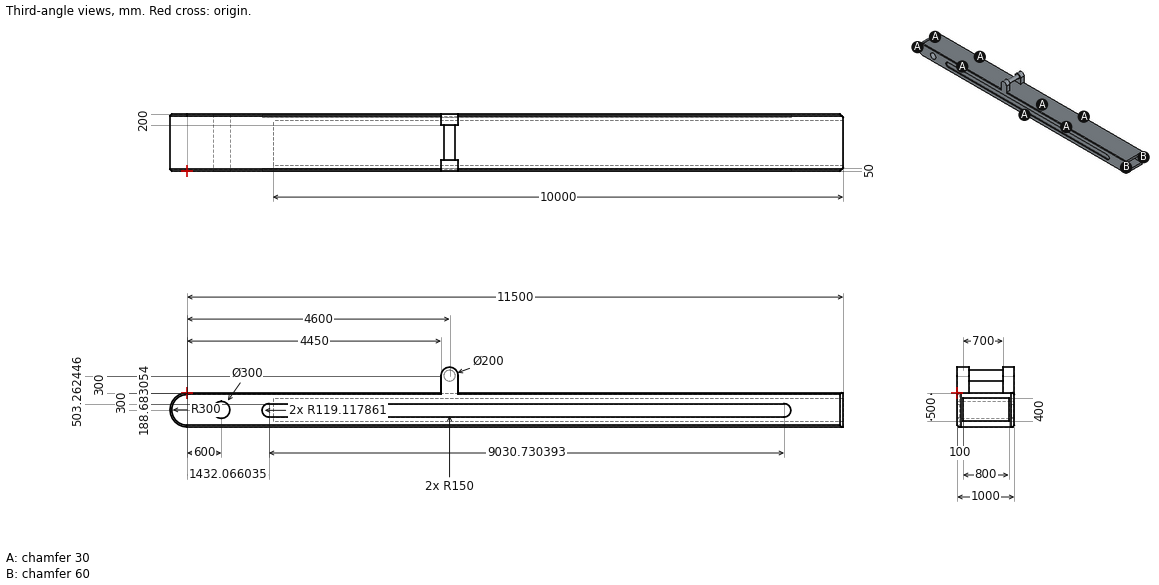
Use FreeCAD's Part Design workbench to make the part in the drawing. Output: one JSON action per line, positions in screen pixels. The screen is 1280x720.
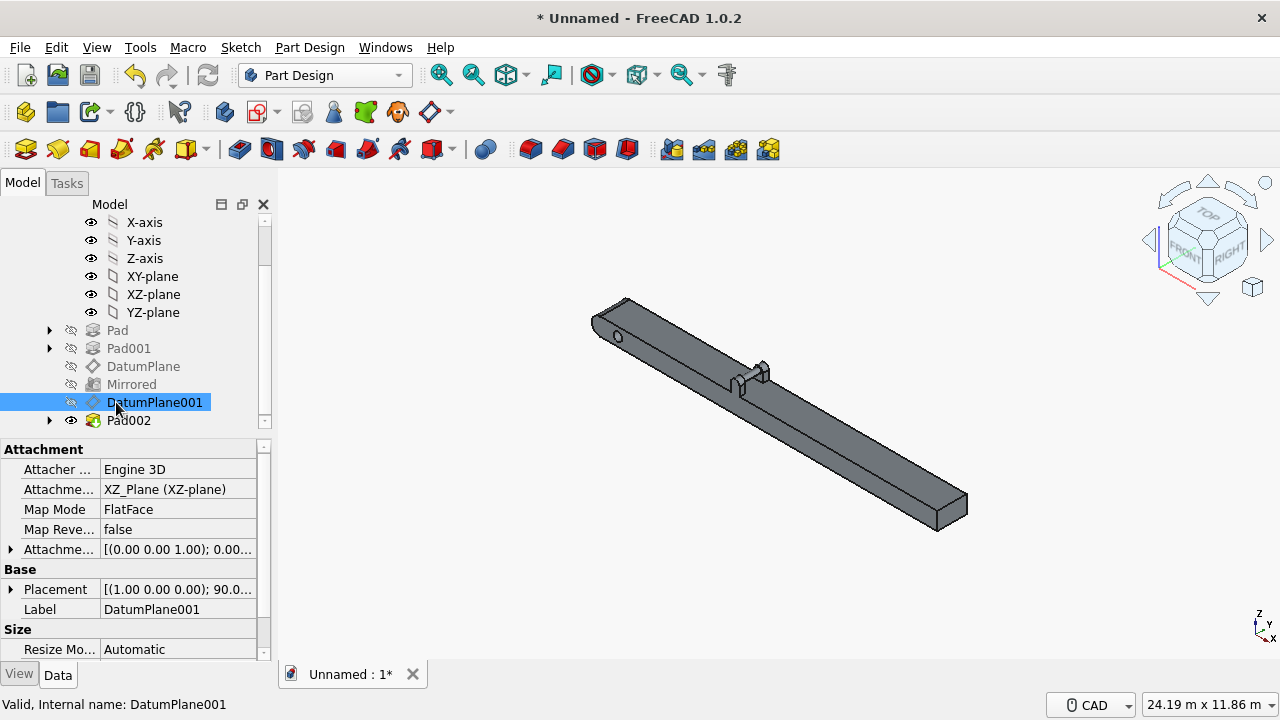
{"action": "left_click", "coordinate": [952, 512]}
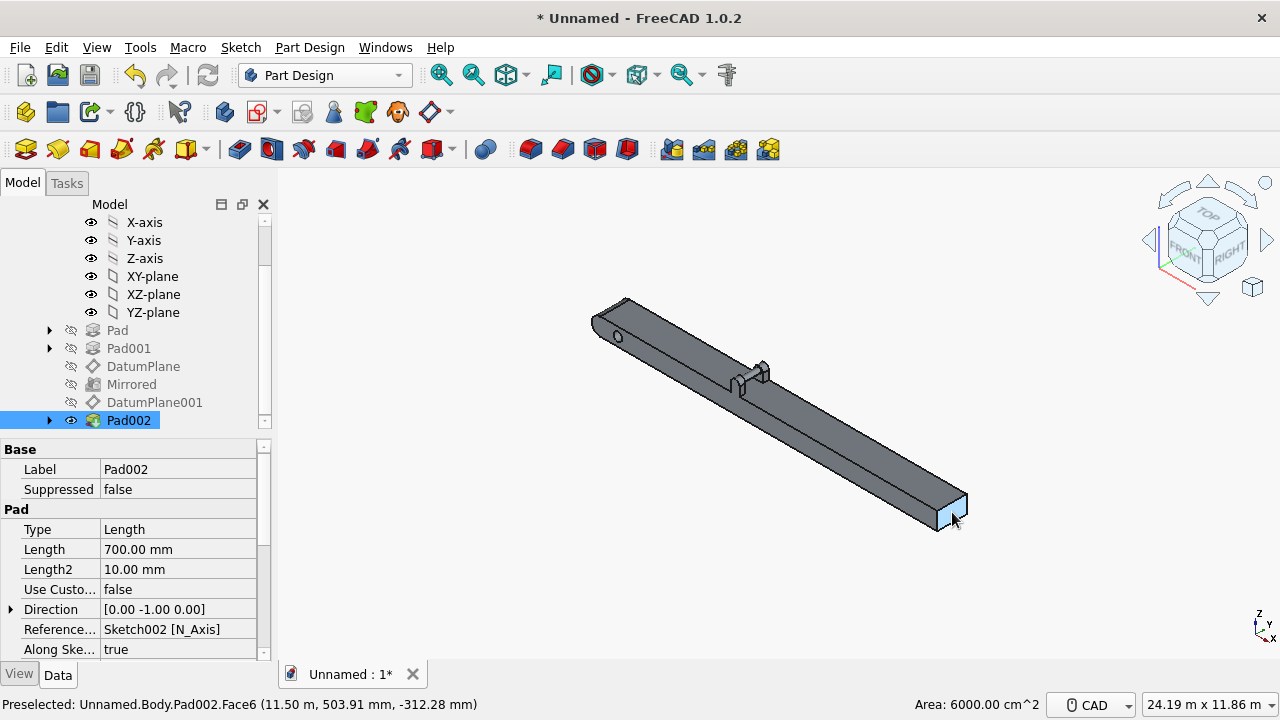
{"action": "left_click", "coordinate": [258, 112]}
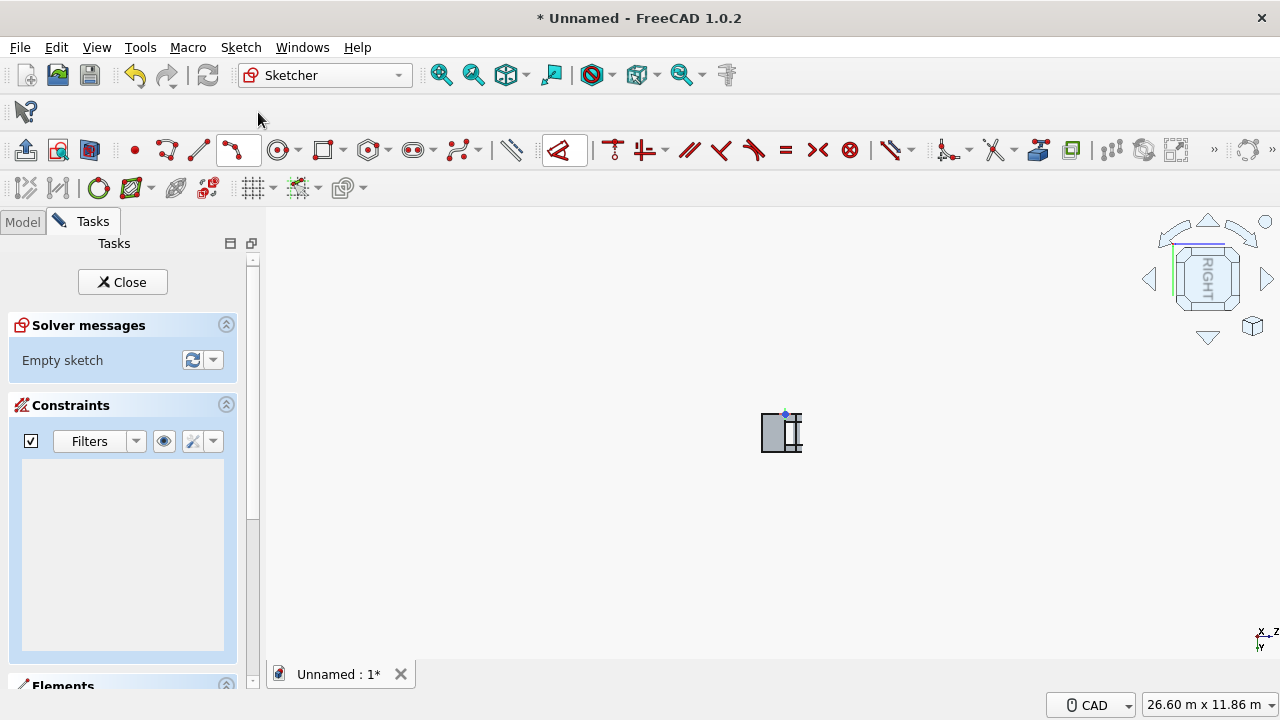
{"action": "scroll", "coordinate": [787, 431], "scroll_direction": "up", "scroll_amount": 10}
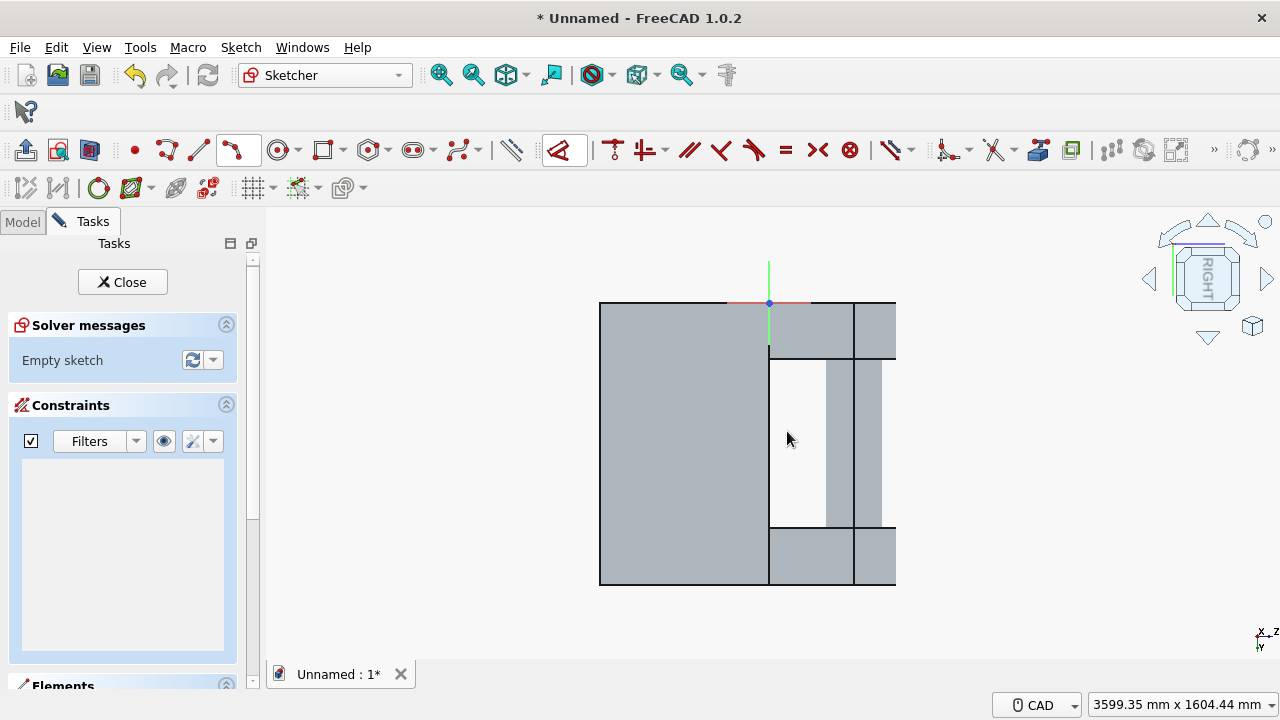
{"action": "left_click", "coordinate": [324, 150]}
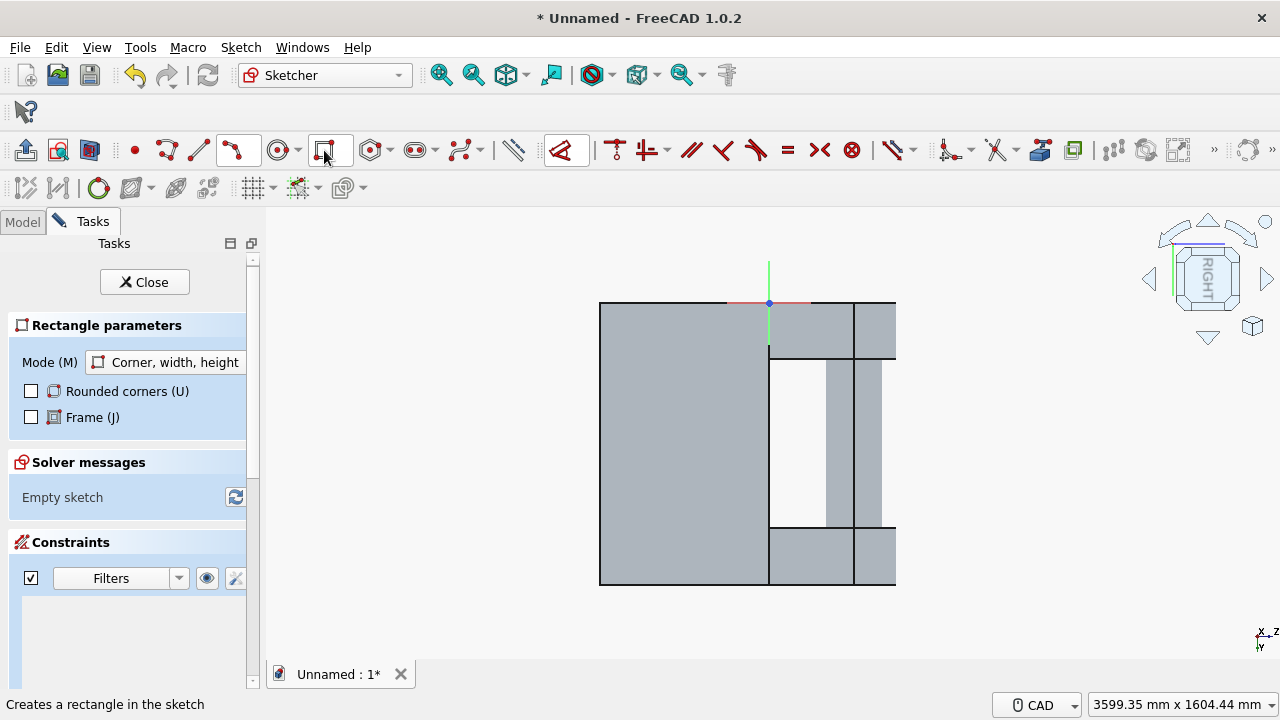
{"action": "left_click", "coordinate": [628, 331]}
{"action": "left_click", "coordinate": [741, 557]}
{"action": "key", "text": "Escape"}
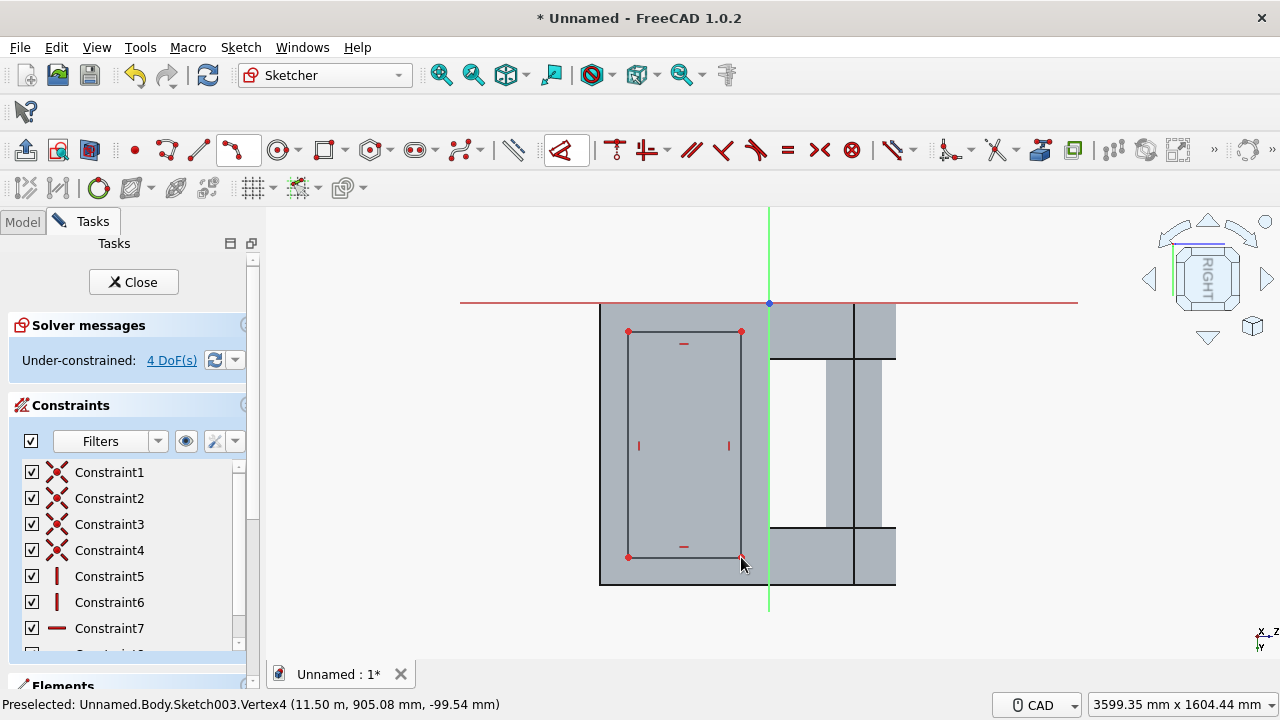
{"action": "left_click", "coordinate": [628, 400]}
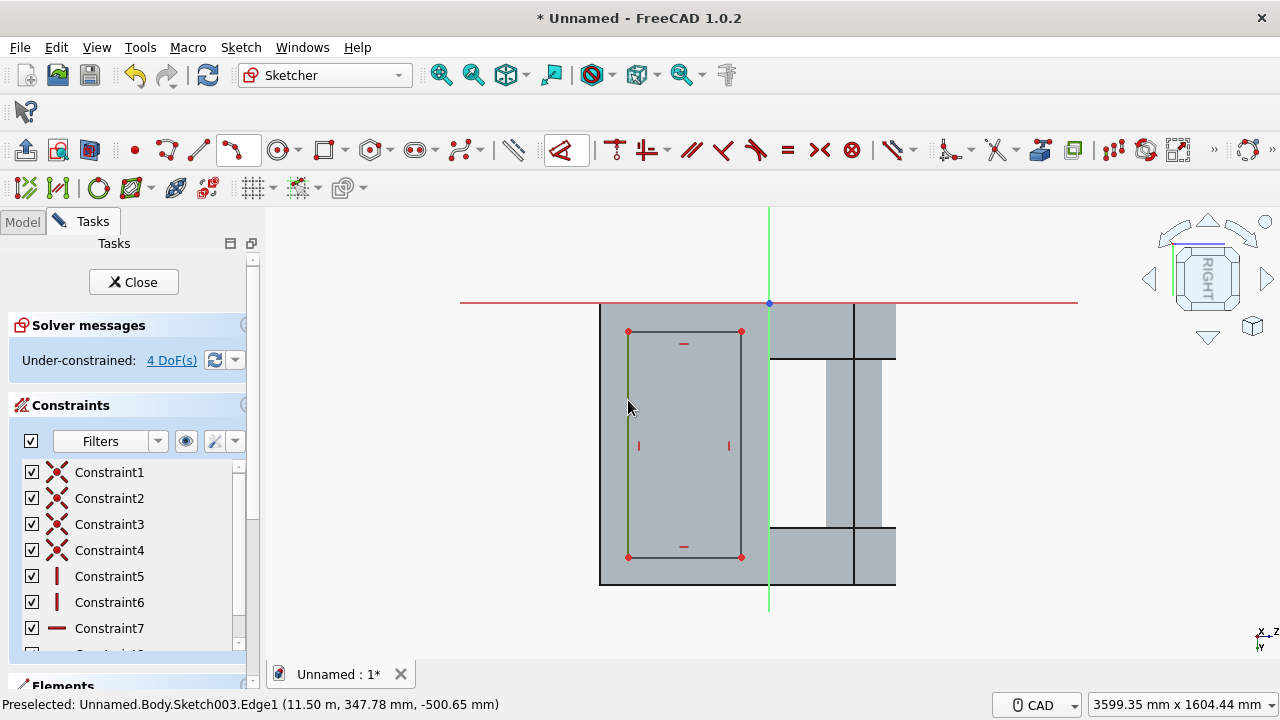
{"action": "key", "text": "i"}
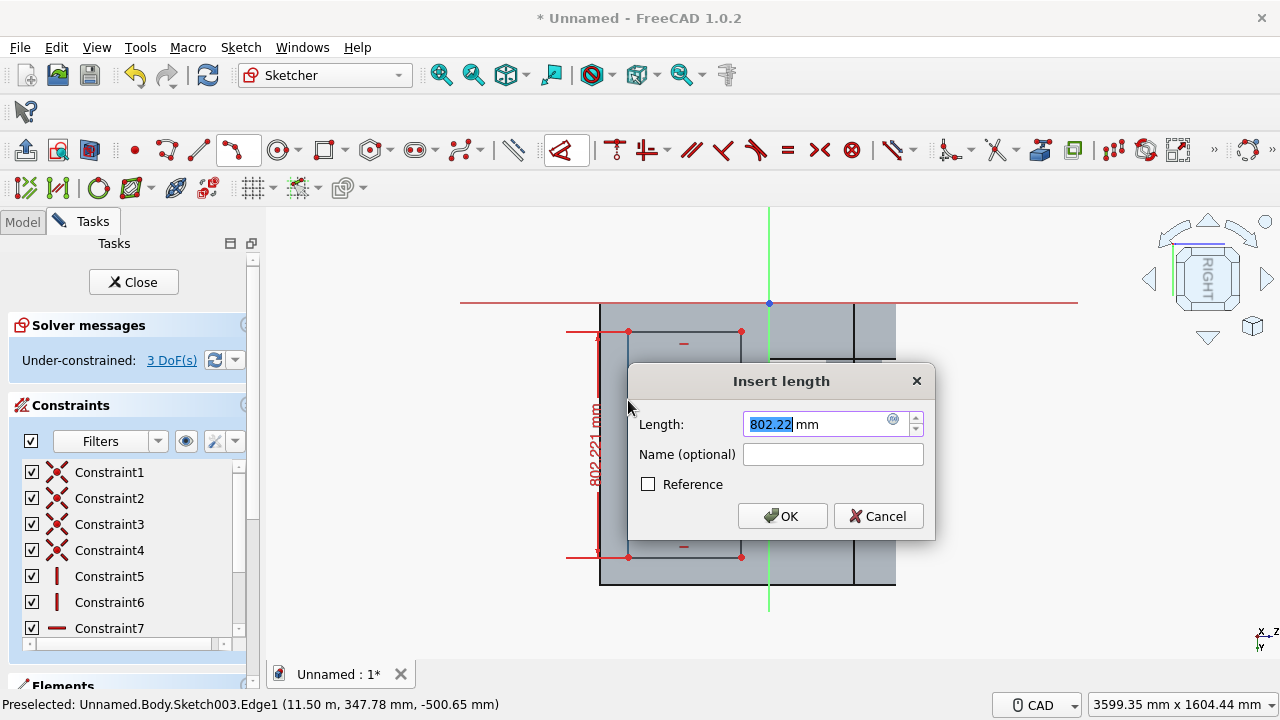
{"action": "type", "text": "800"}
{"action": "key", "text": "Return"}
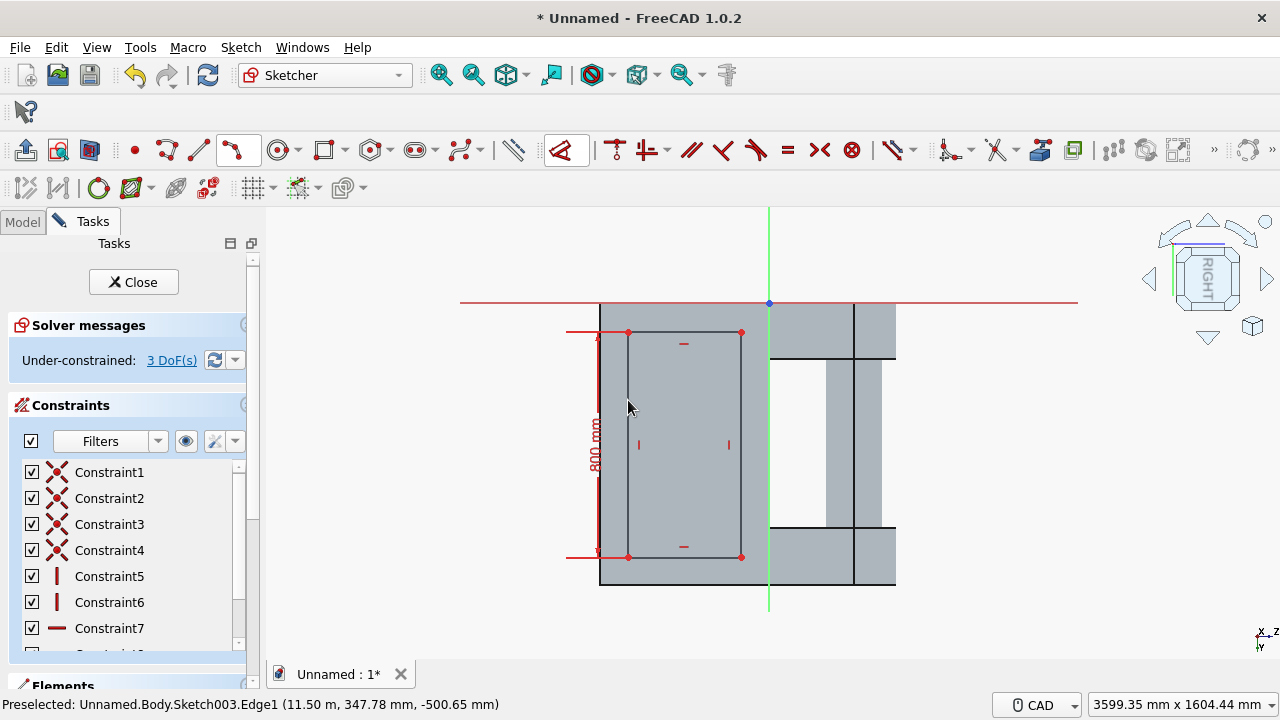
{"action": "left_click", "coordinate": [662, 558]}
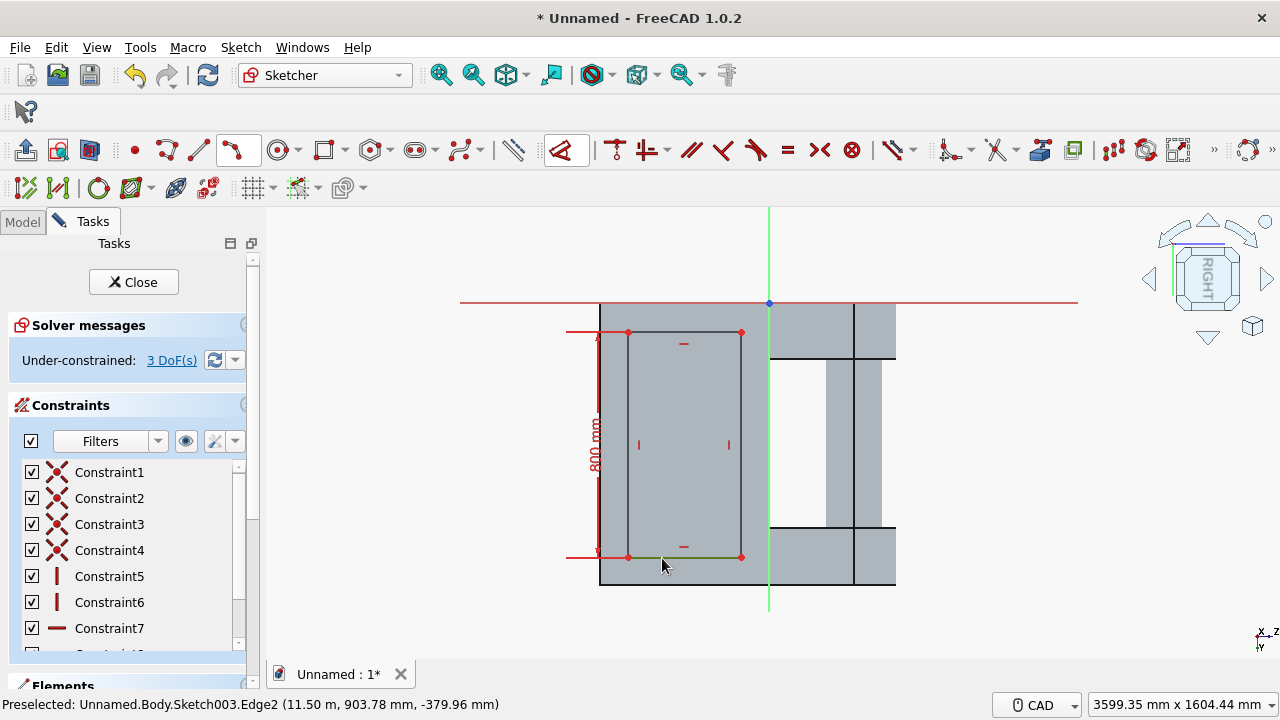
{"action": "left_click", "coordinate": [584, 150]}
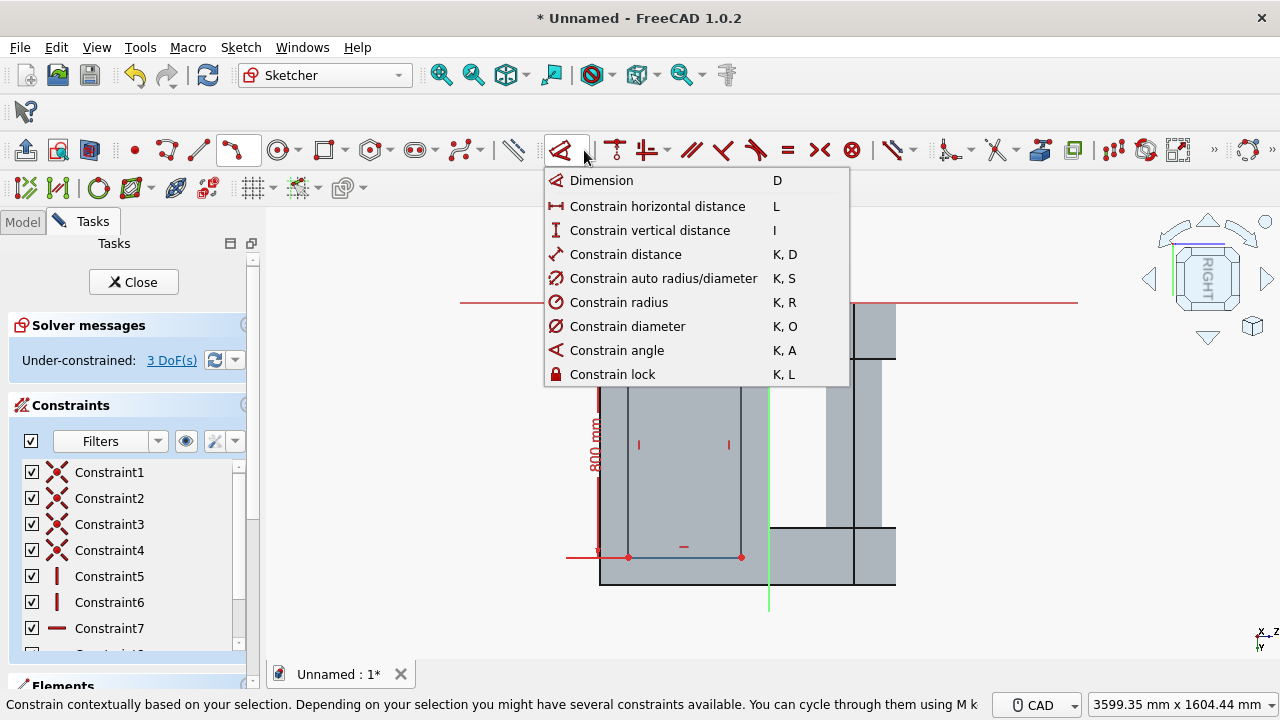
{"action": "left_click", "coordinate": [697, 206]}